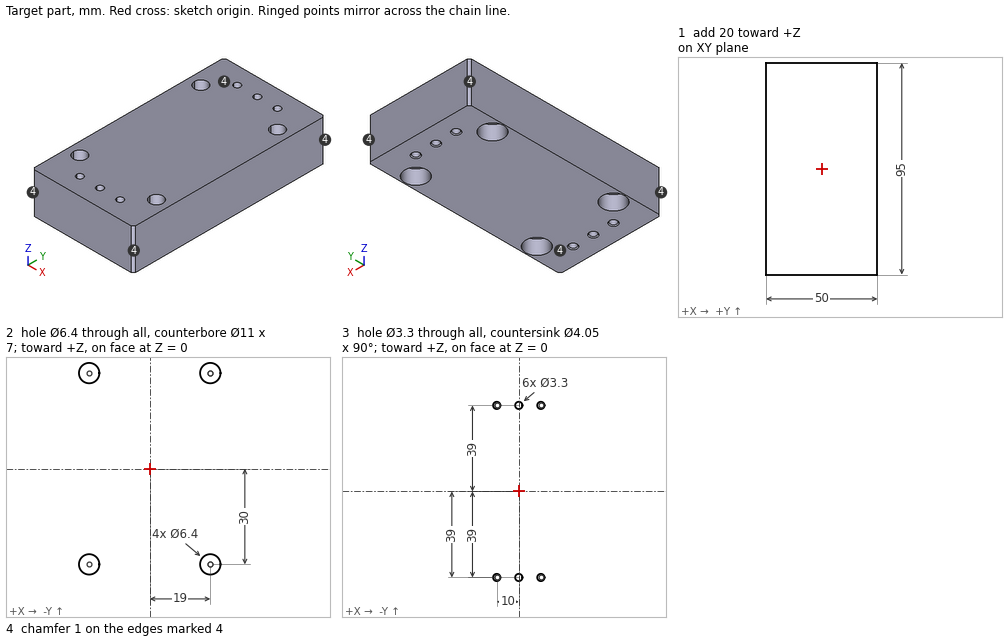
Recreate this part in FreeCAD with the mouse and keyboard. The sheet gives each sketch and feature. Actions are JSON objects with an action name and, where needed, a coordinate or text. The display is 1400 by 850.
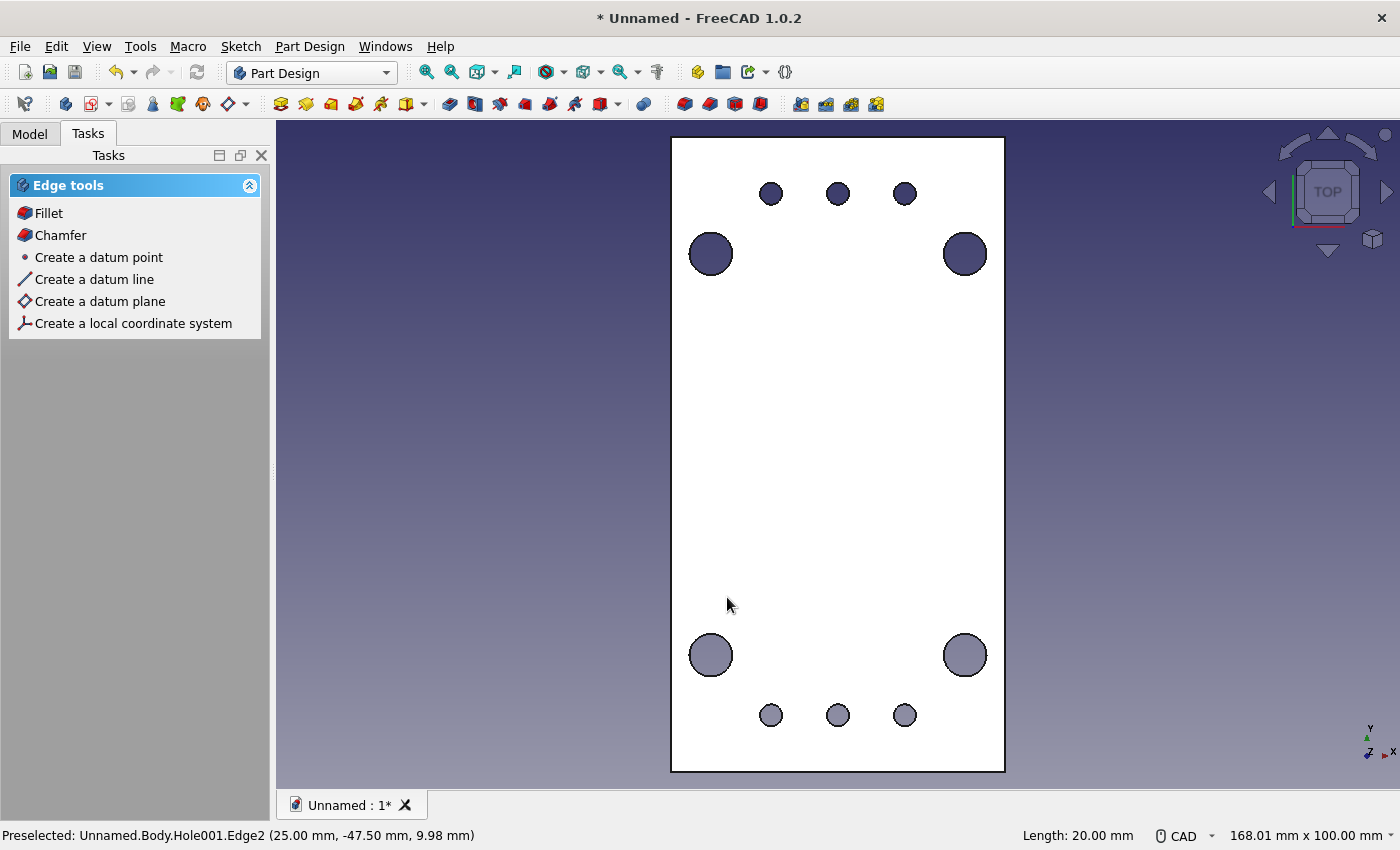
{"action": "key", "text": "1"}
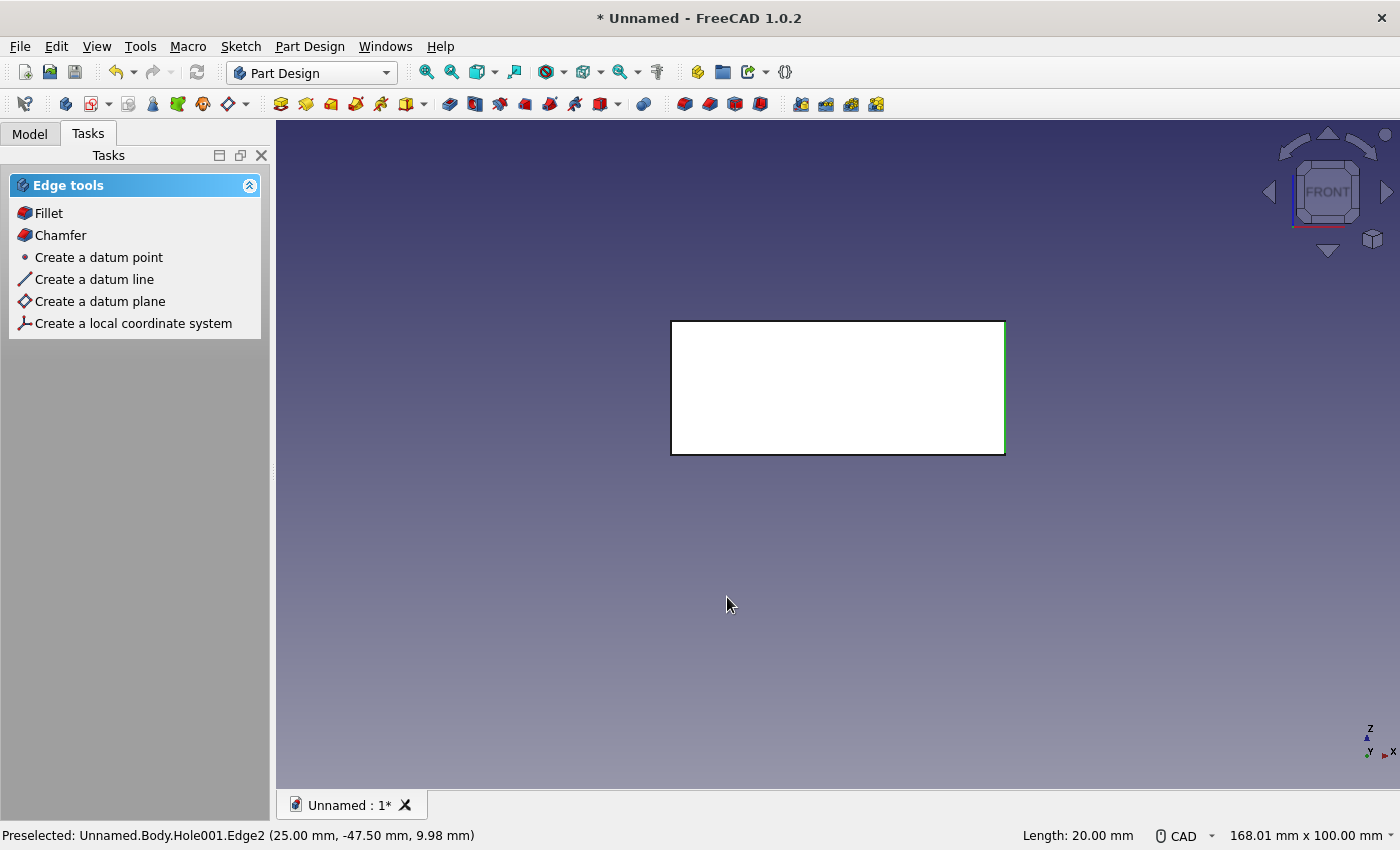
{"action": "left_click", "coordinate": [427, 72]}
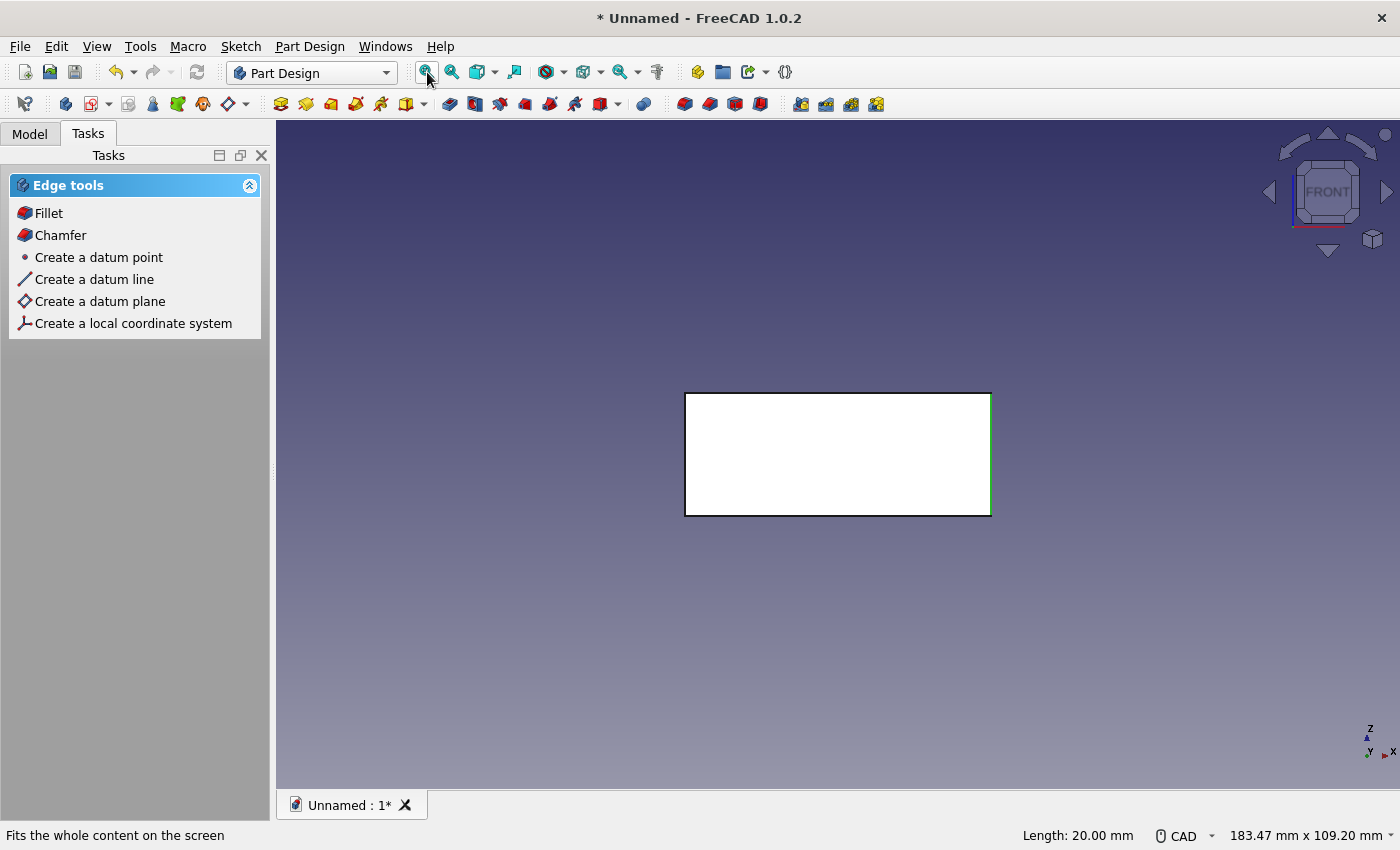
{"action": "left_click", "coordinate": [685, 454], "text": "ctrl"}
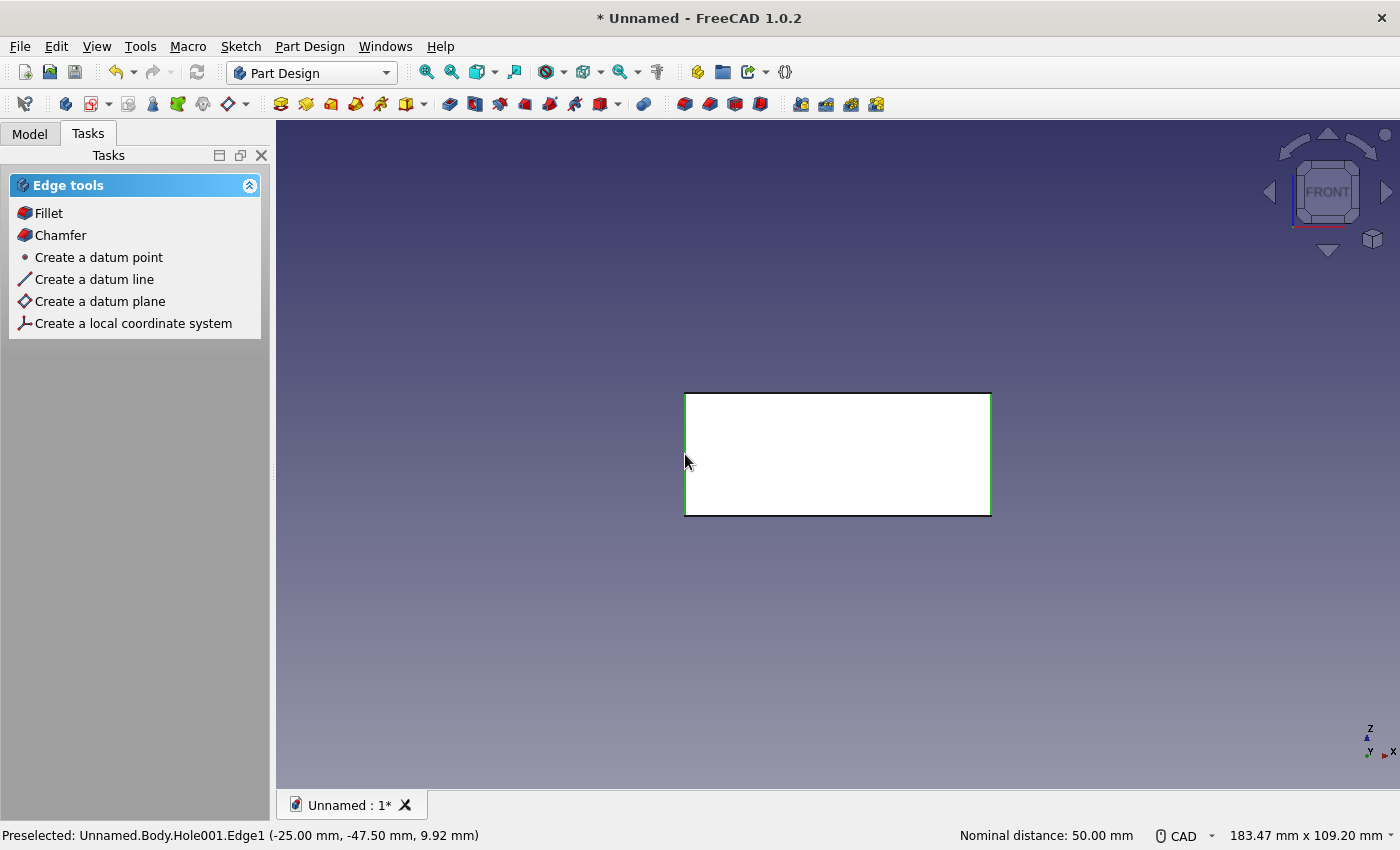
{"action": "key", "text": "3"}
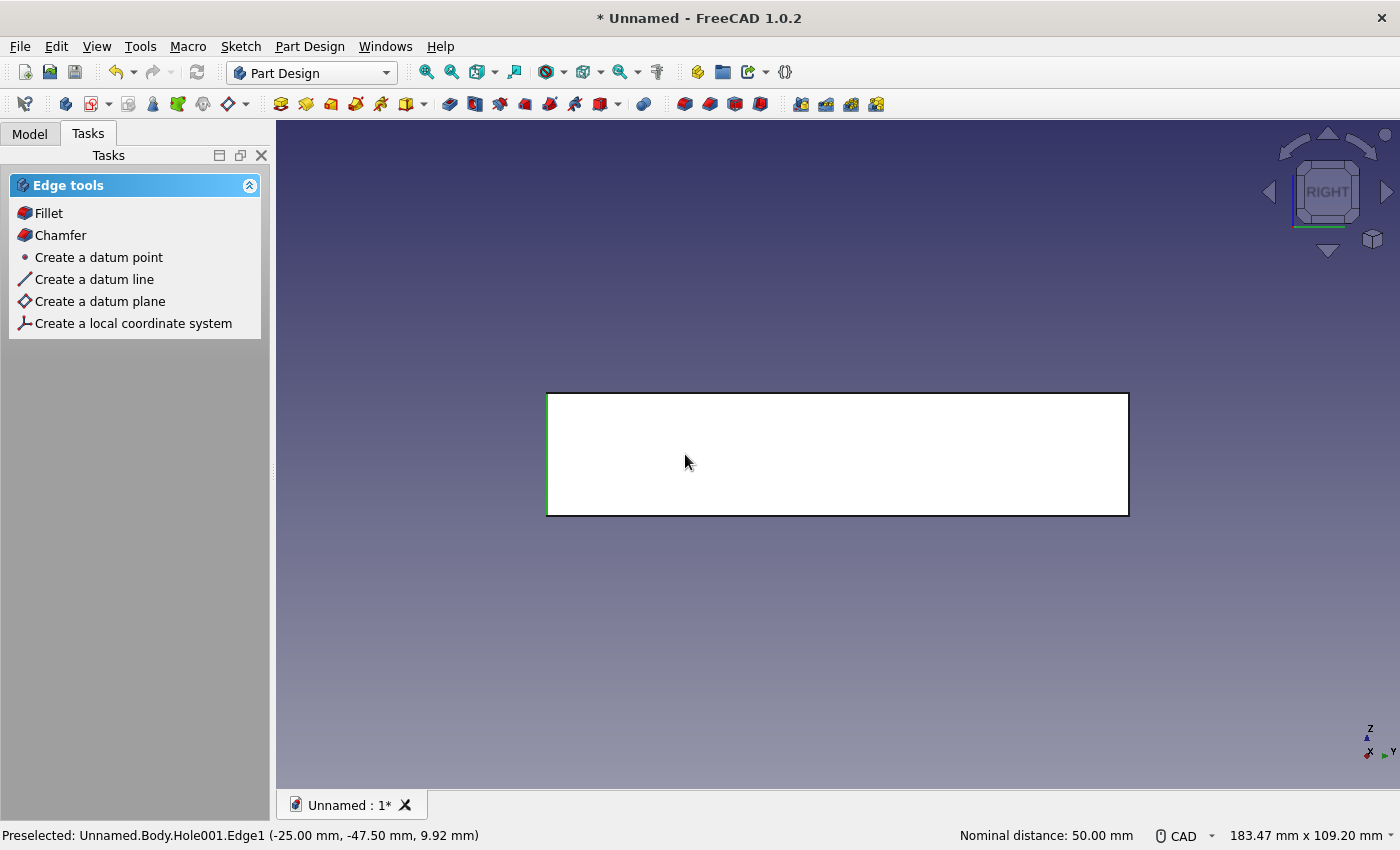
{"action": "left_click", "coordinate": [1129, 453], "text": "ctrl"}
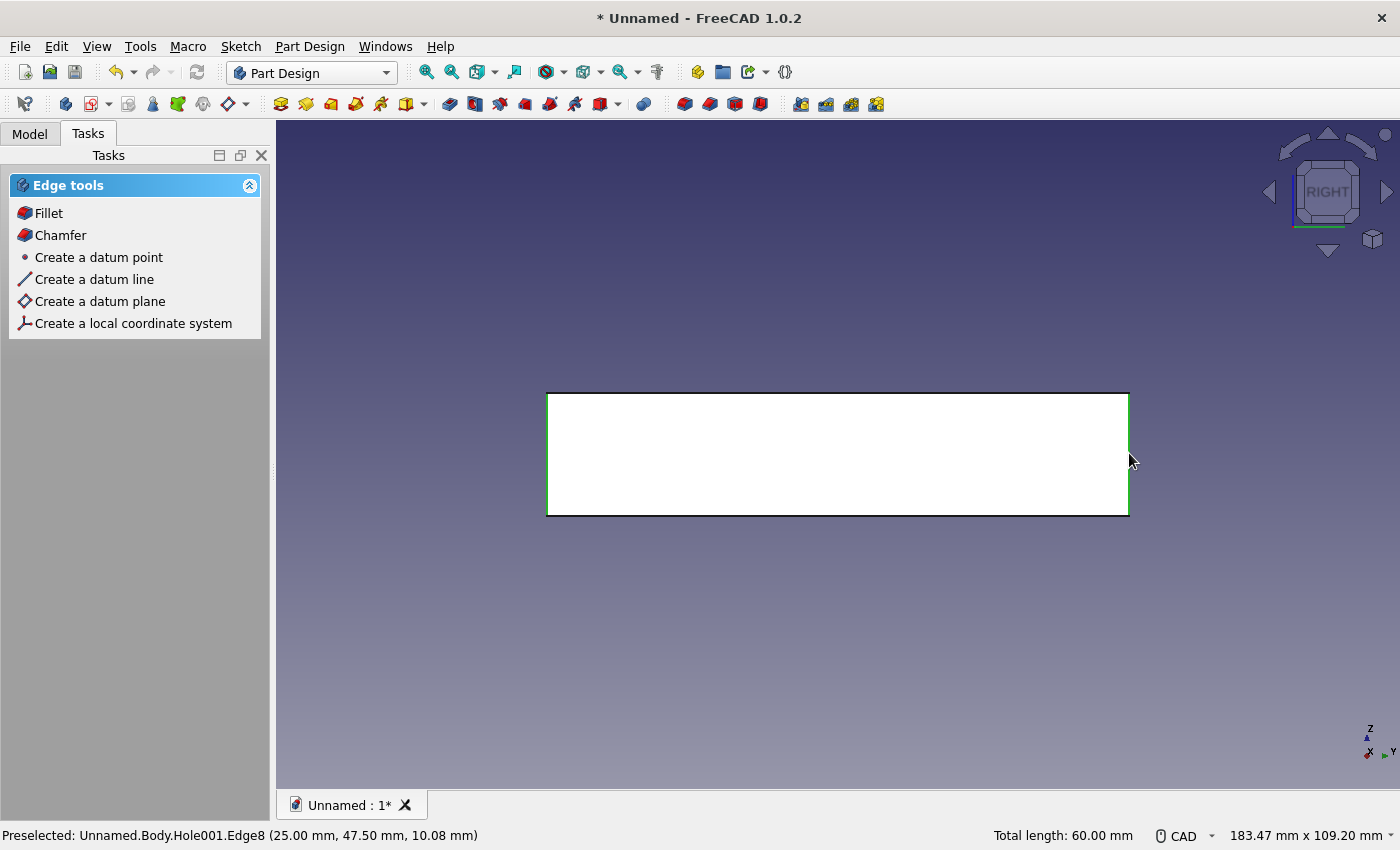
{"action": "key", "text": "5"}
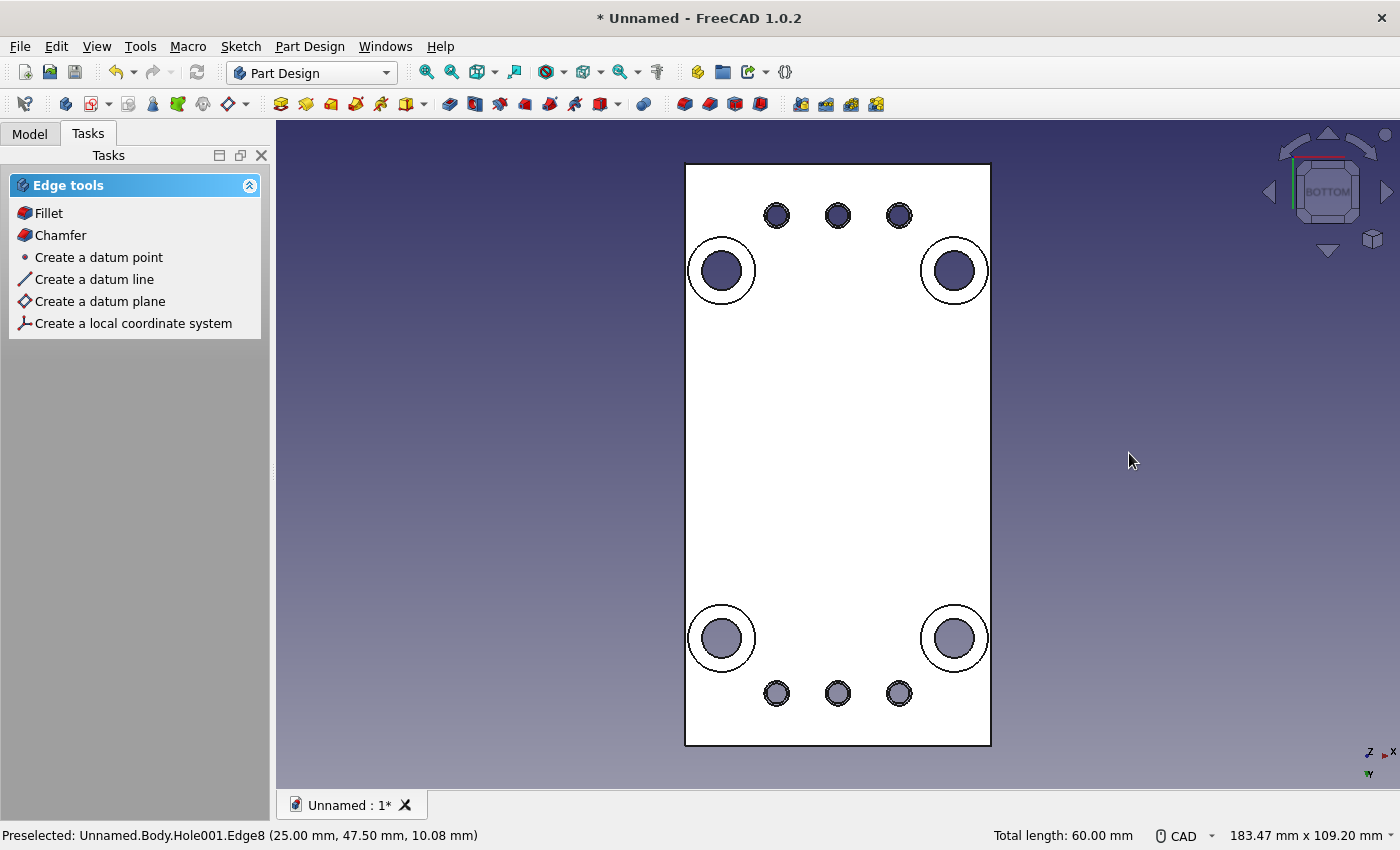
{"action": "key", "text": "4"}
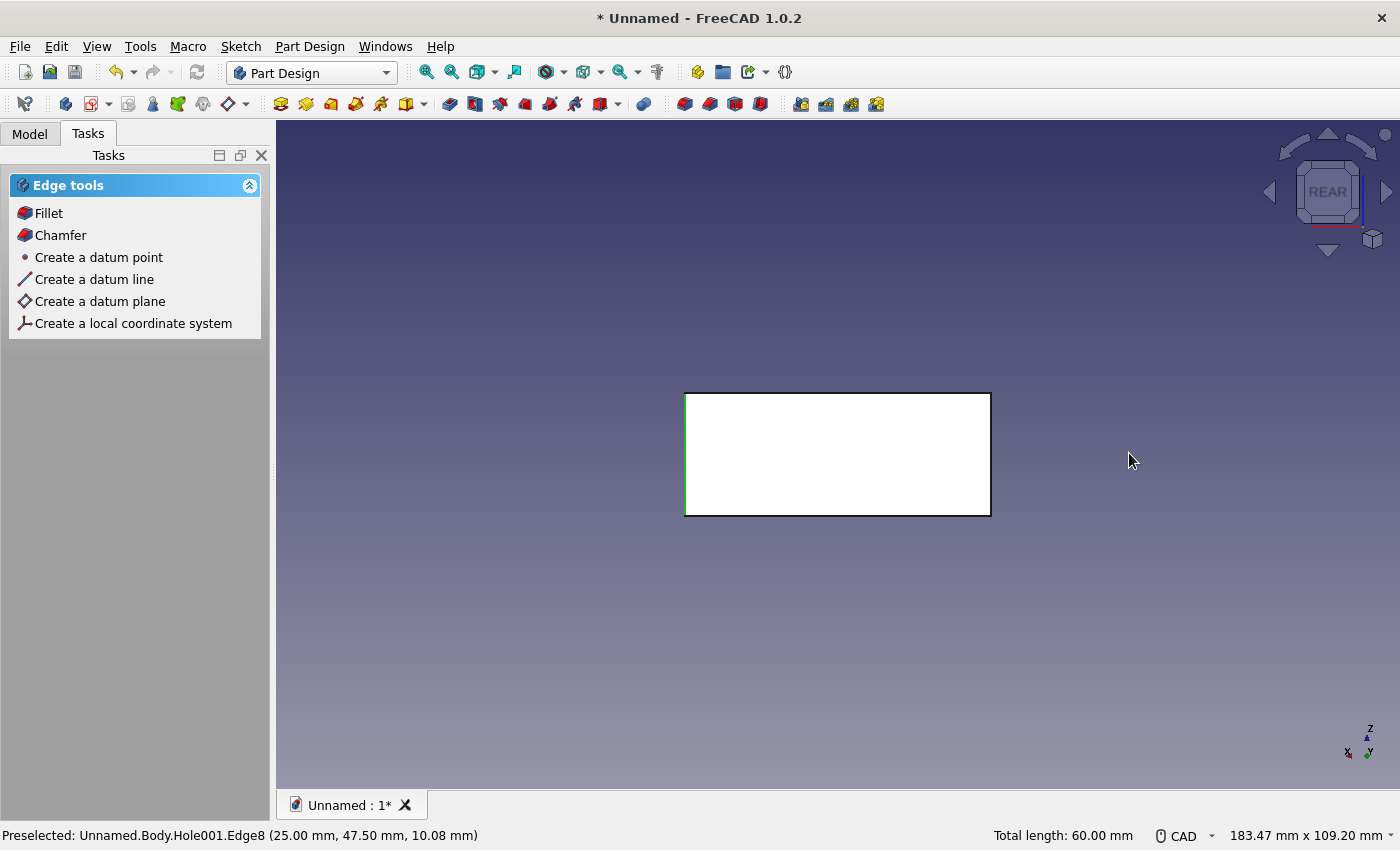
{"action": "left_click", "coordinate": [427, 72]}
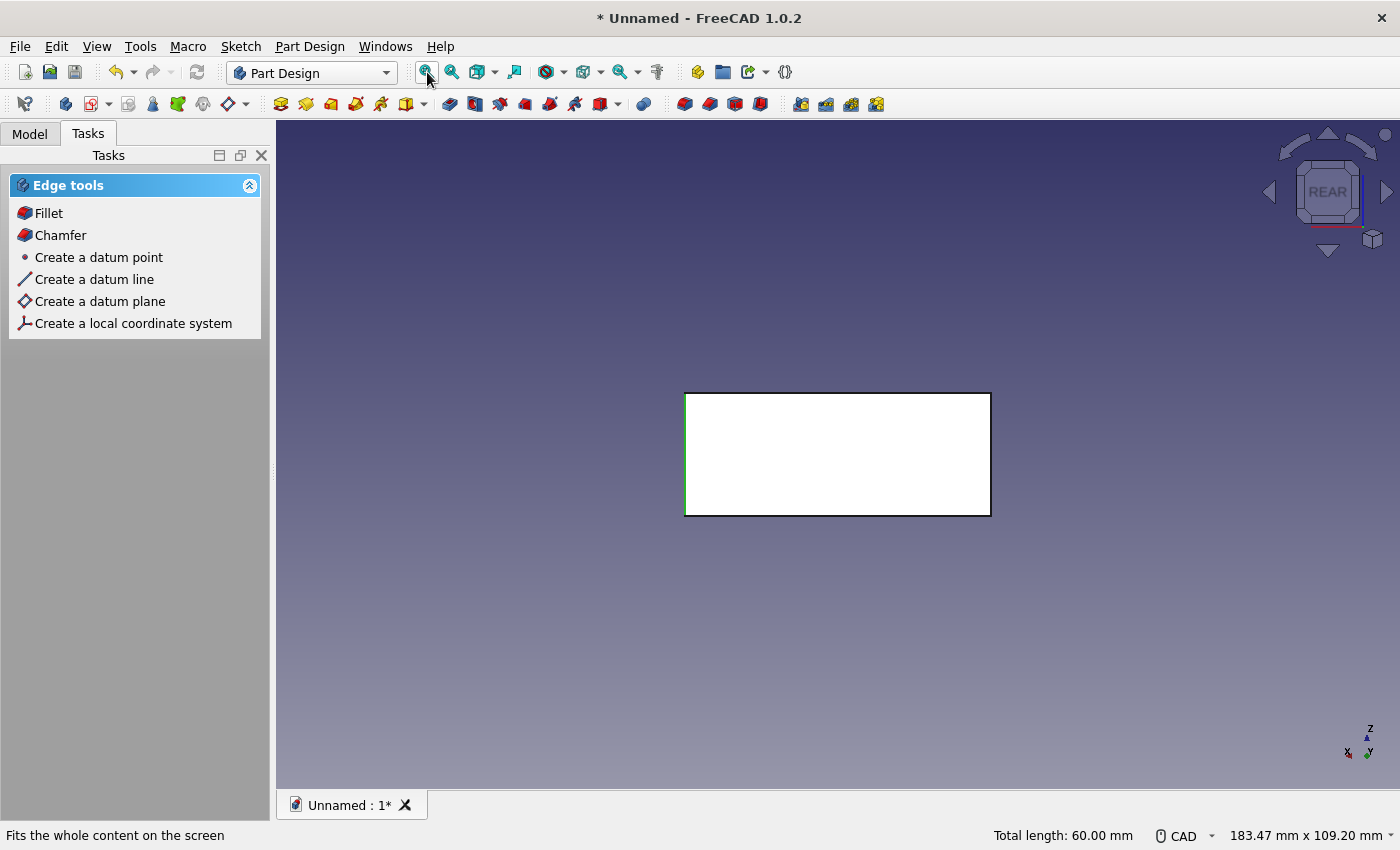
{"action": "left_click", "coordinate": [991, 454], "text": "ctrl"}